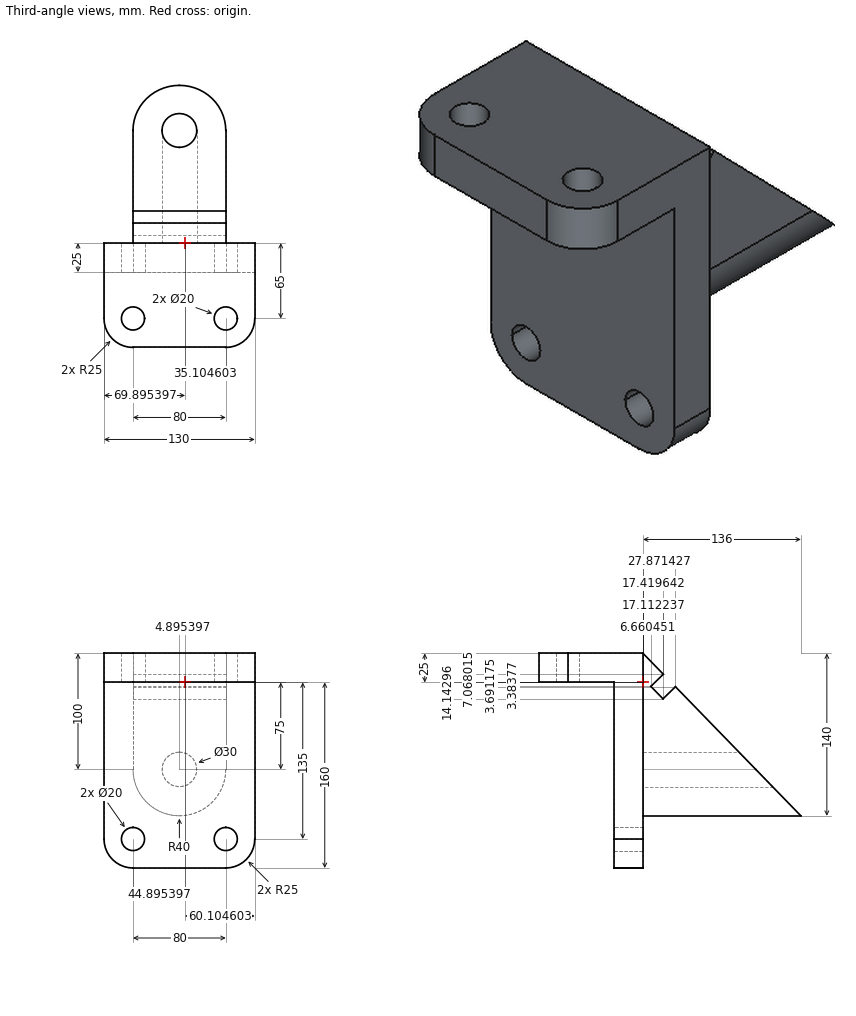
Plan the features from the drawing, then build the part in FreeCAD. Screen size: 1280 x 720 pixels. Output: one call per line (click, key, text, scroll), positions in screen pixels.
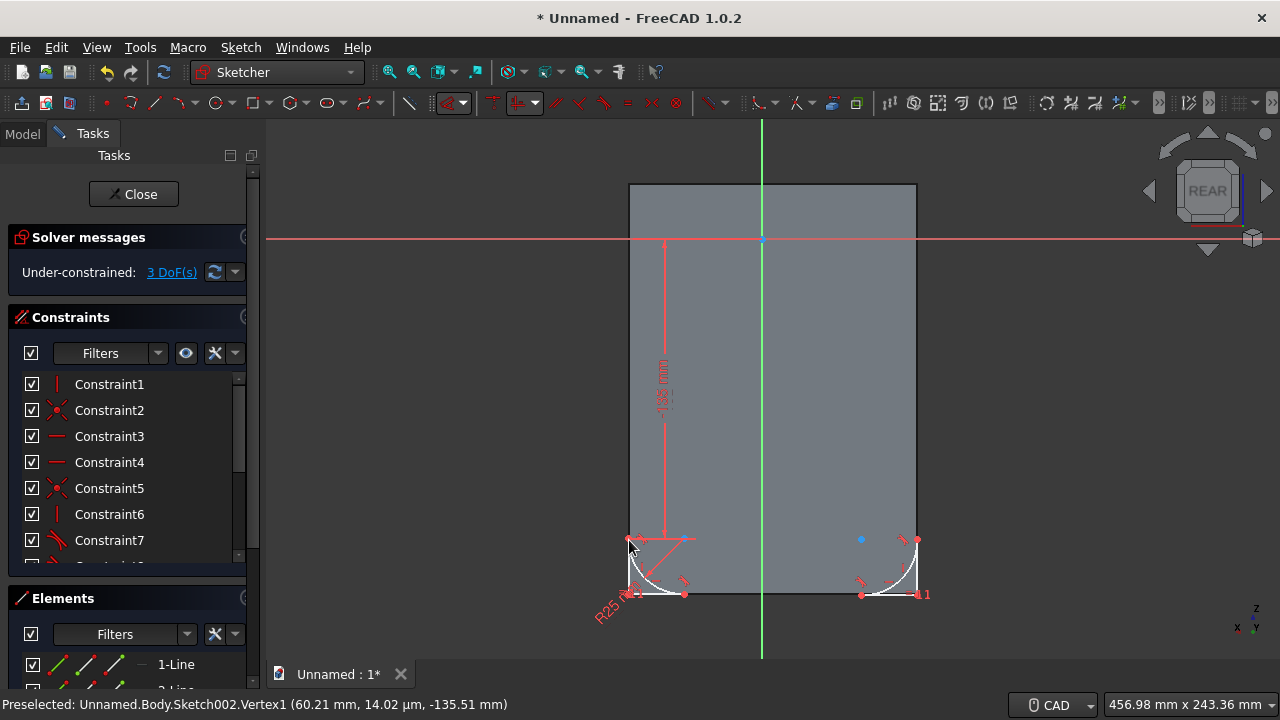
click(862, 595)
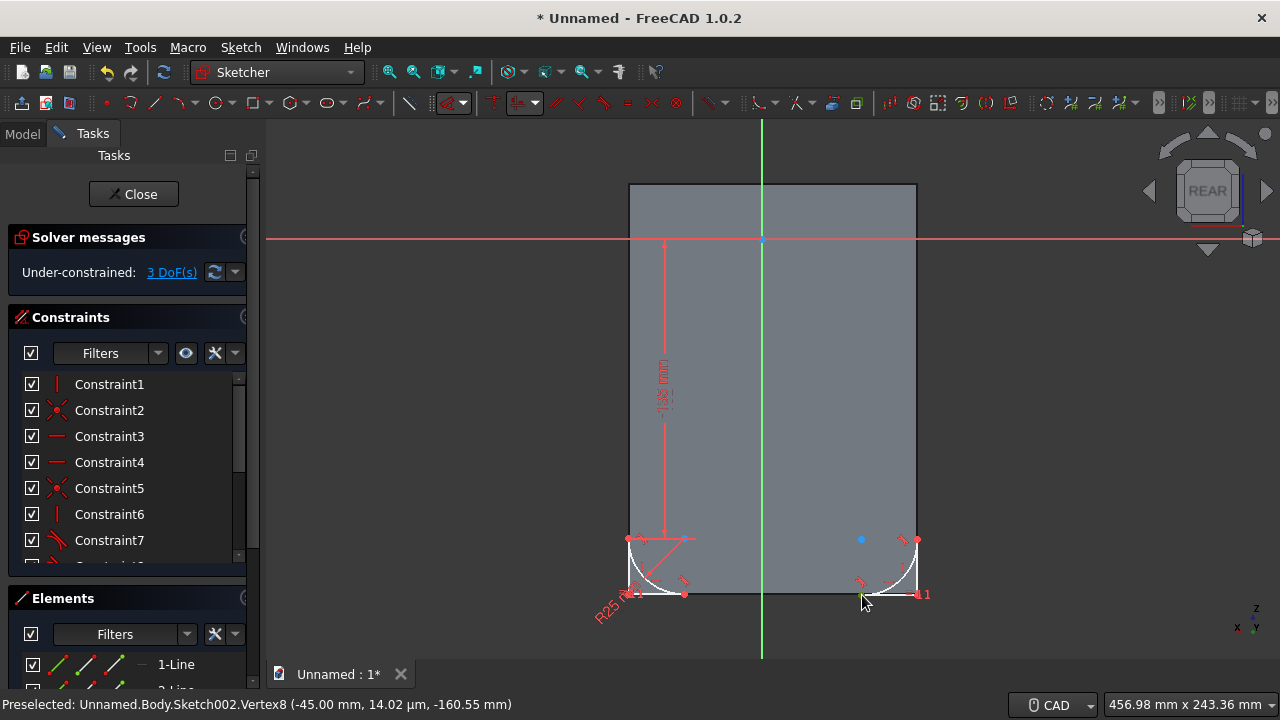
key(i)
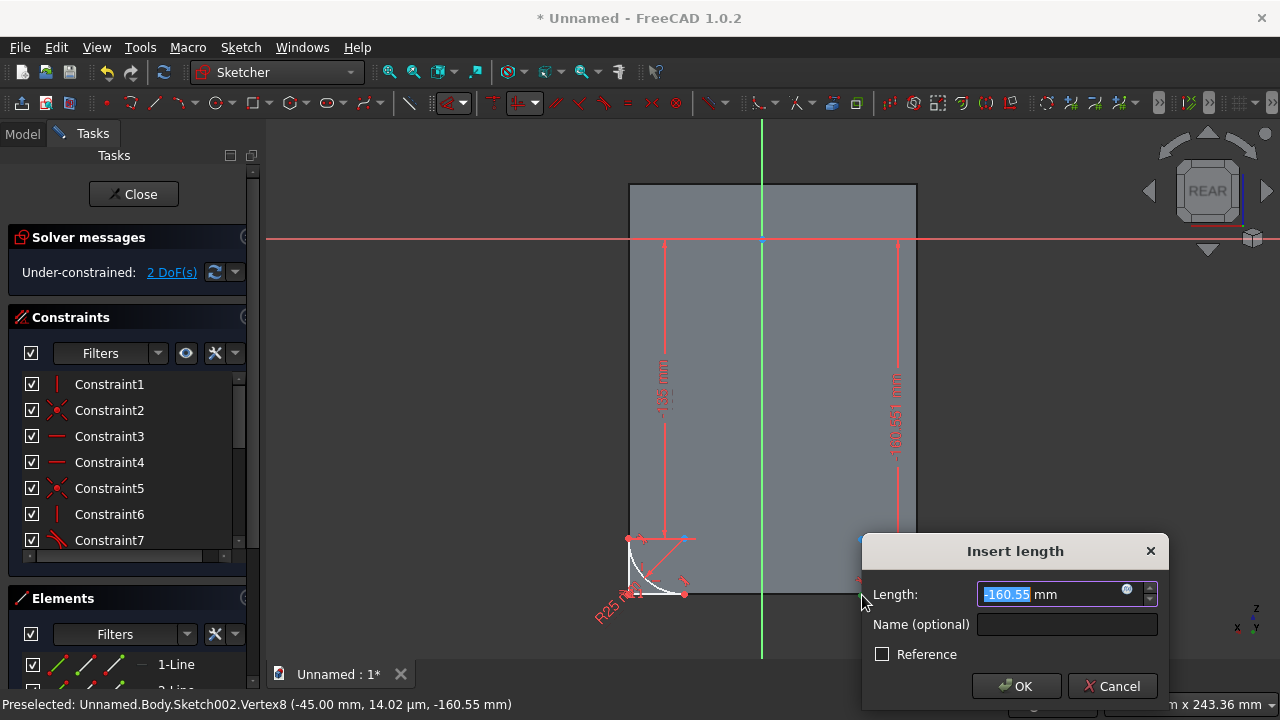
text(-160)
key(Return)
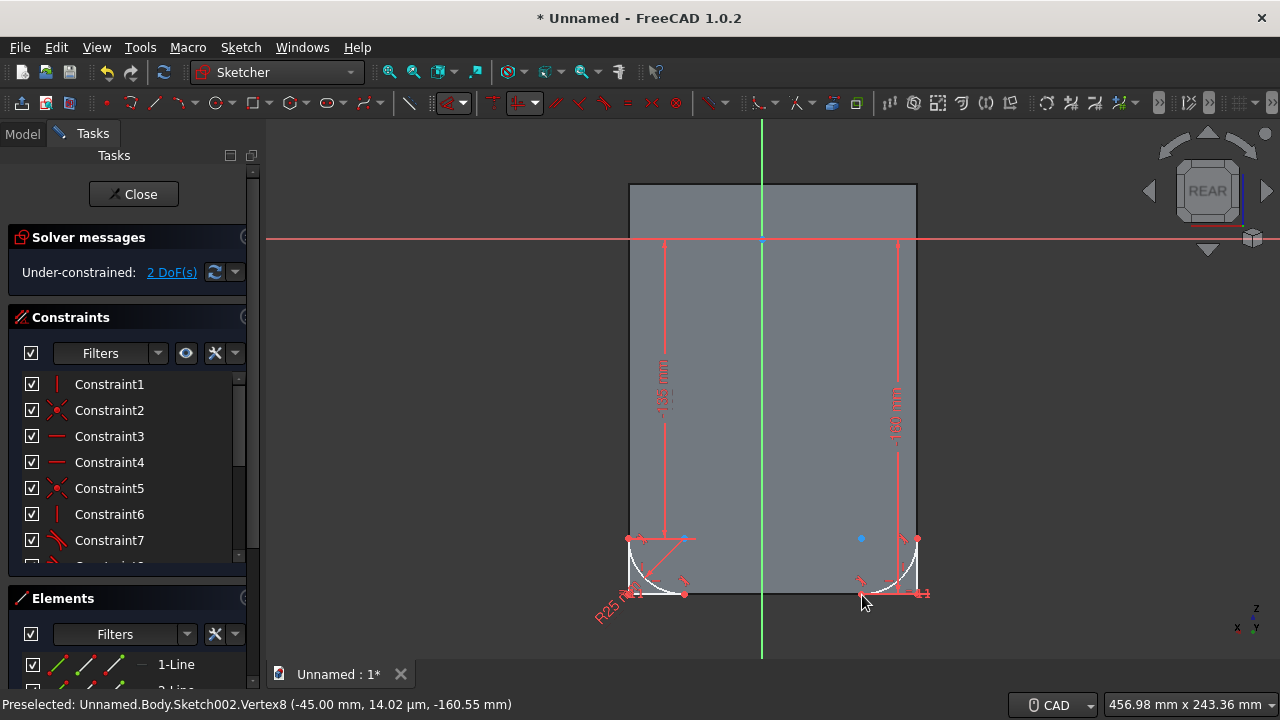
click(629, 539)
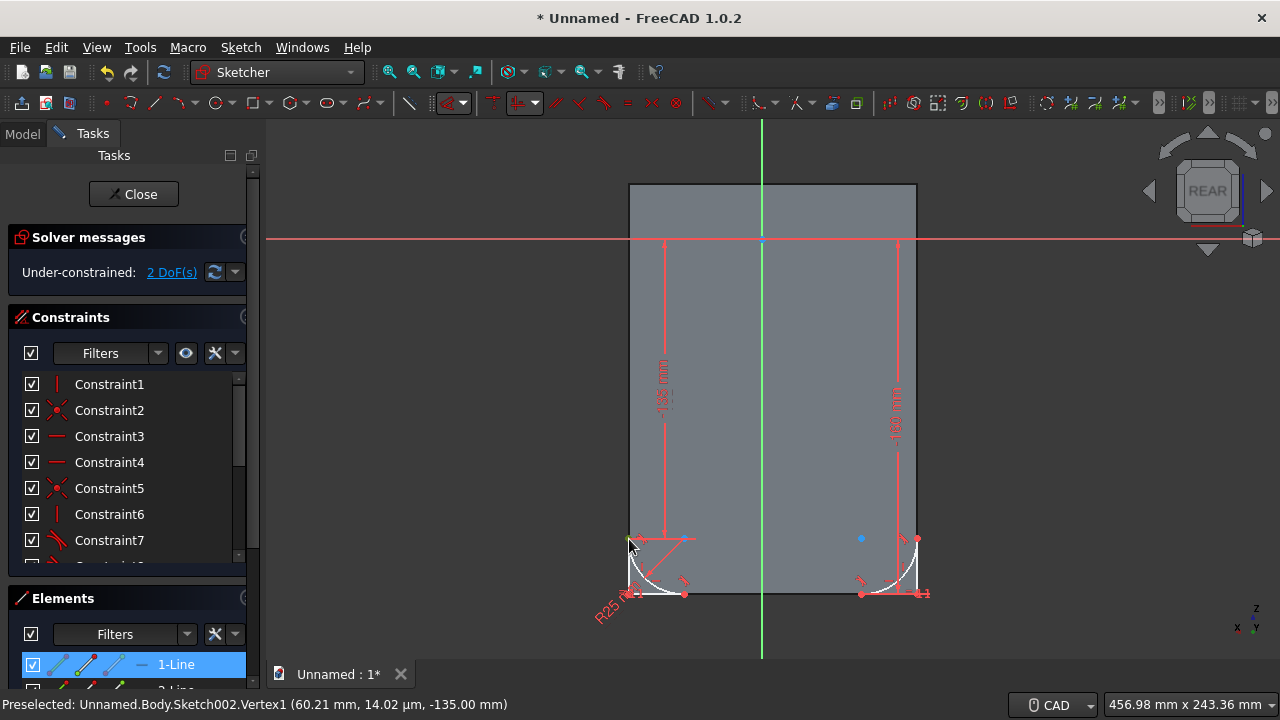
click(466, 104)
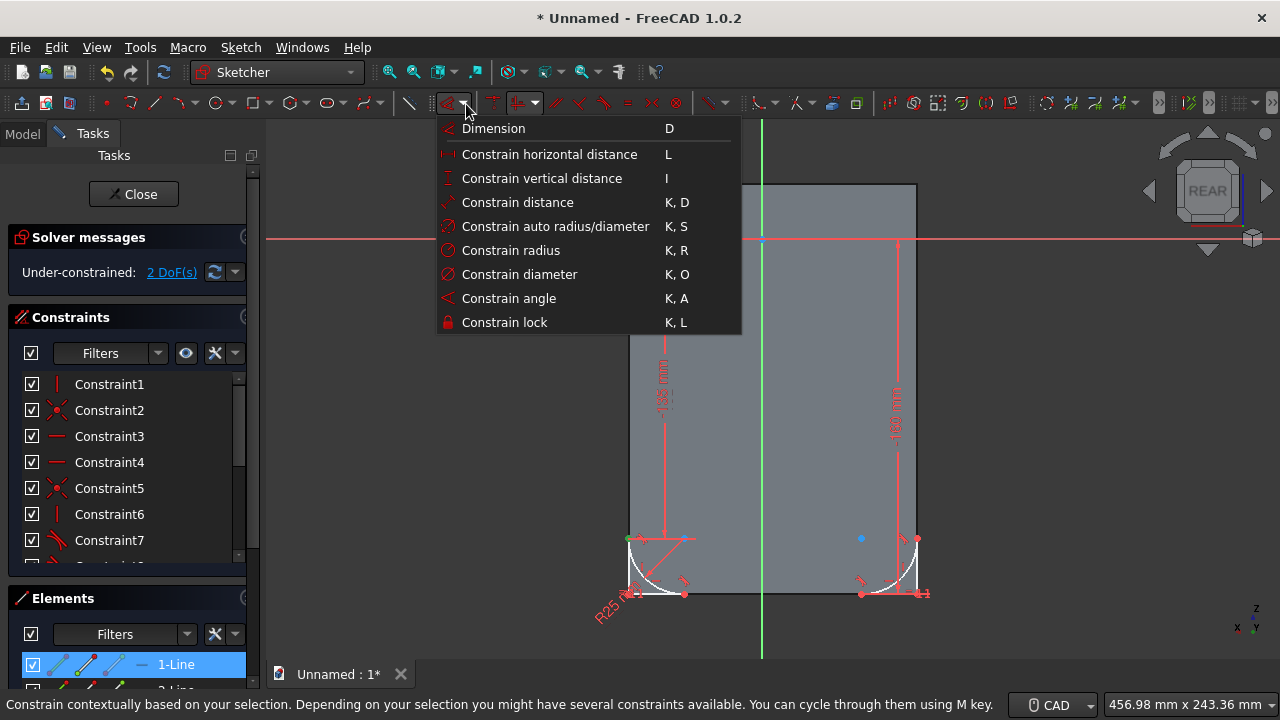
click(589, 154)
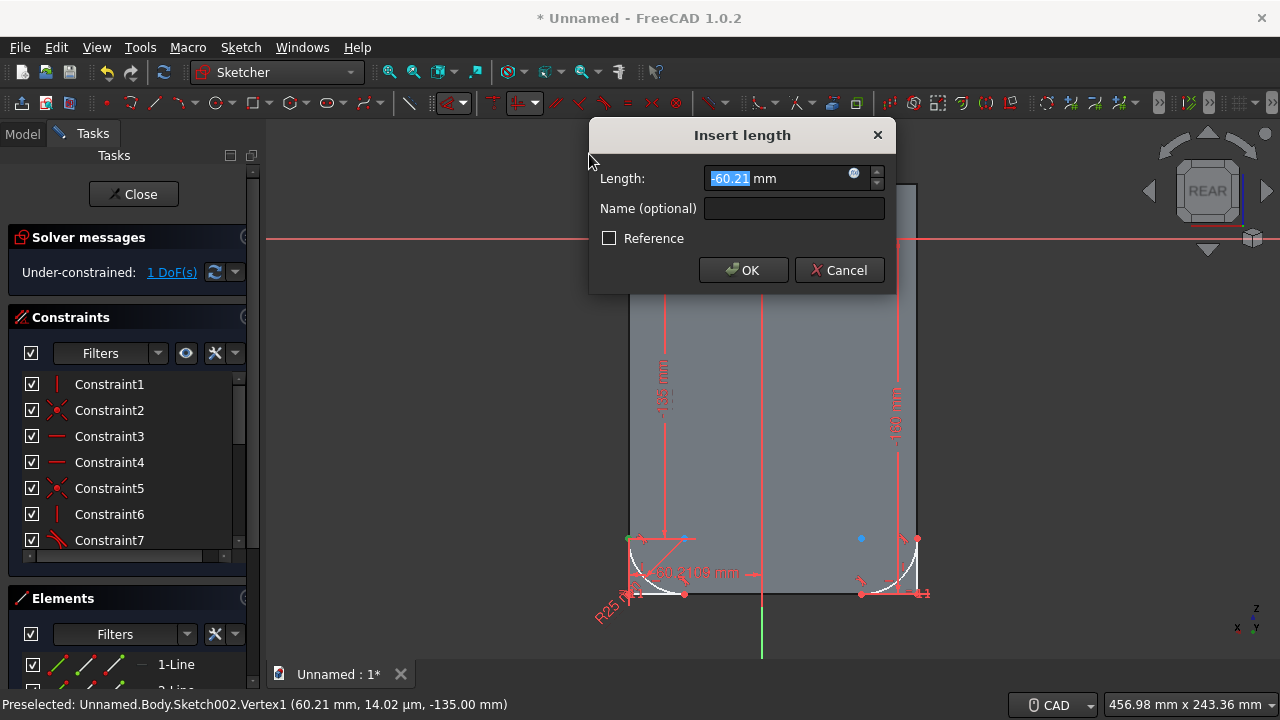
text(-60.104603)
key(Return)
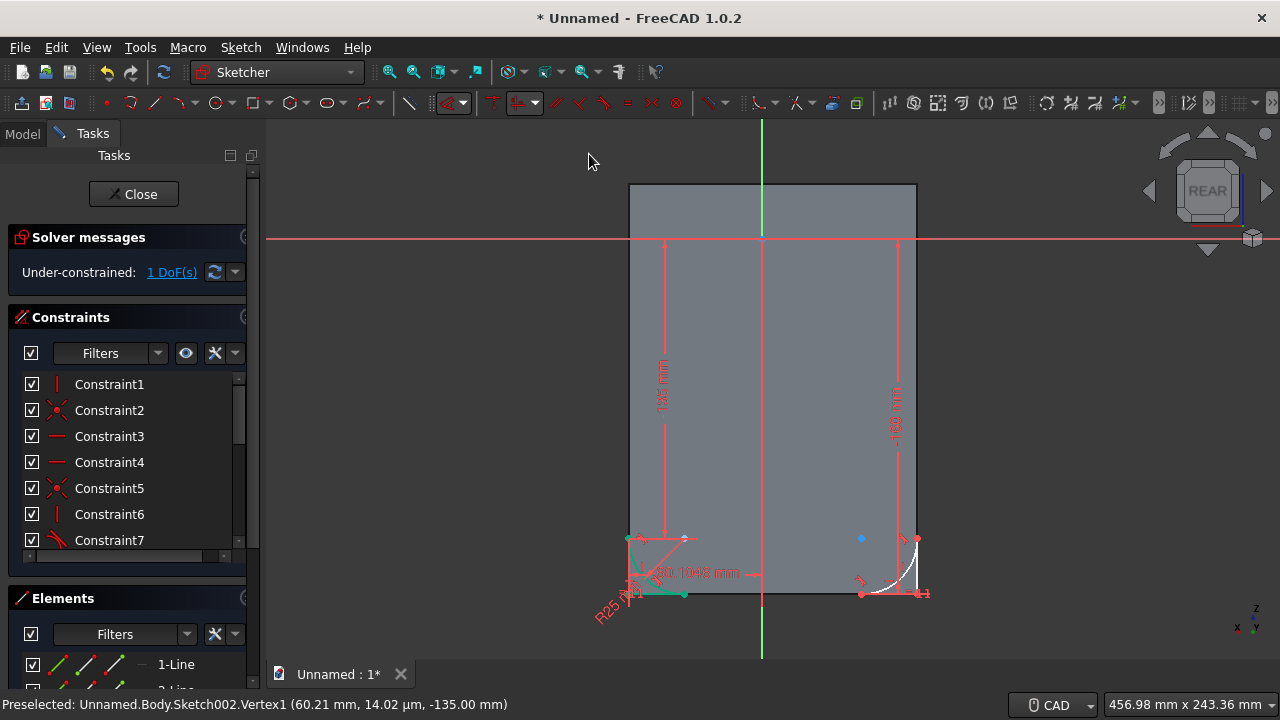
click(862, 594)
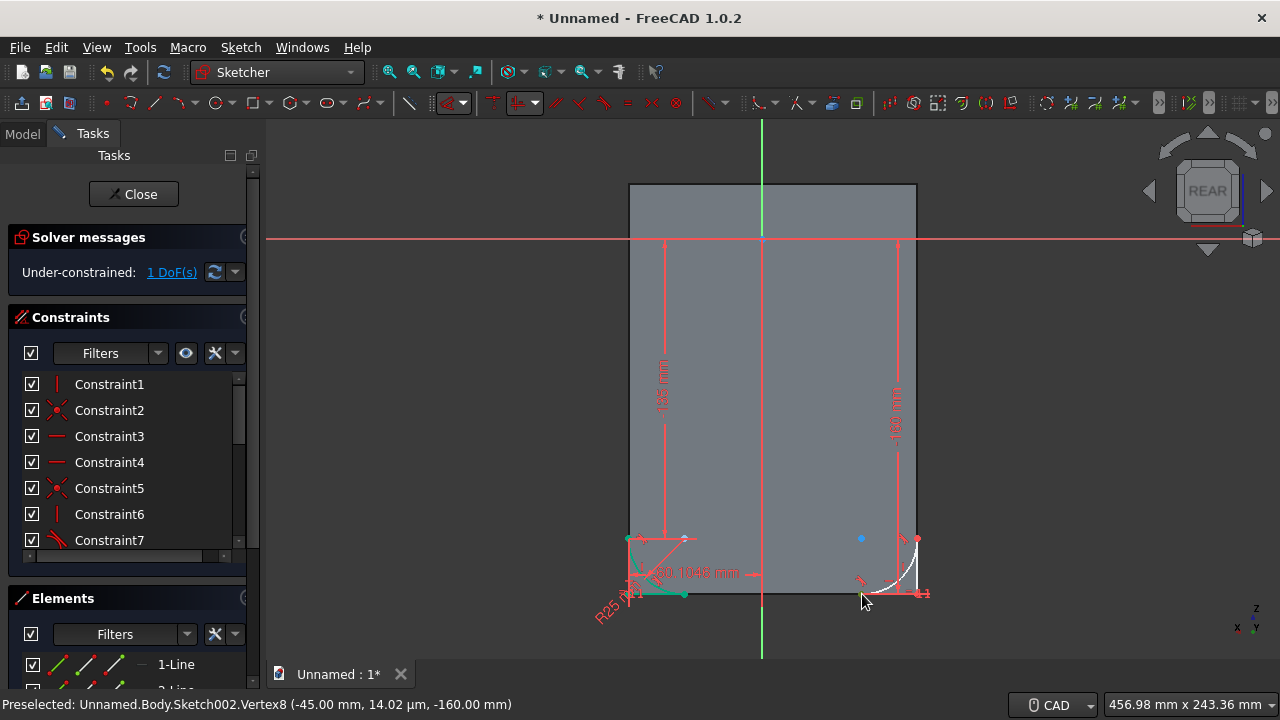
key(l)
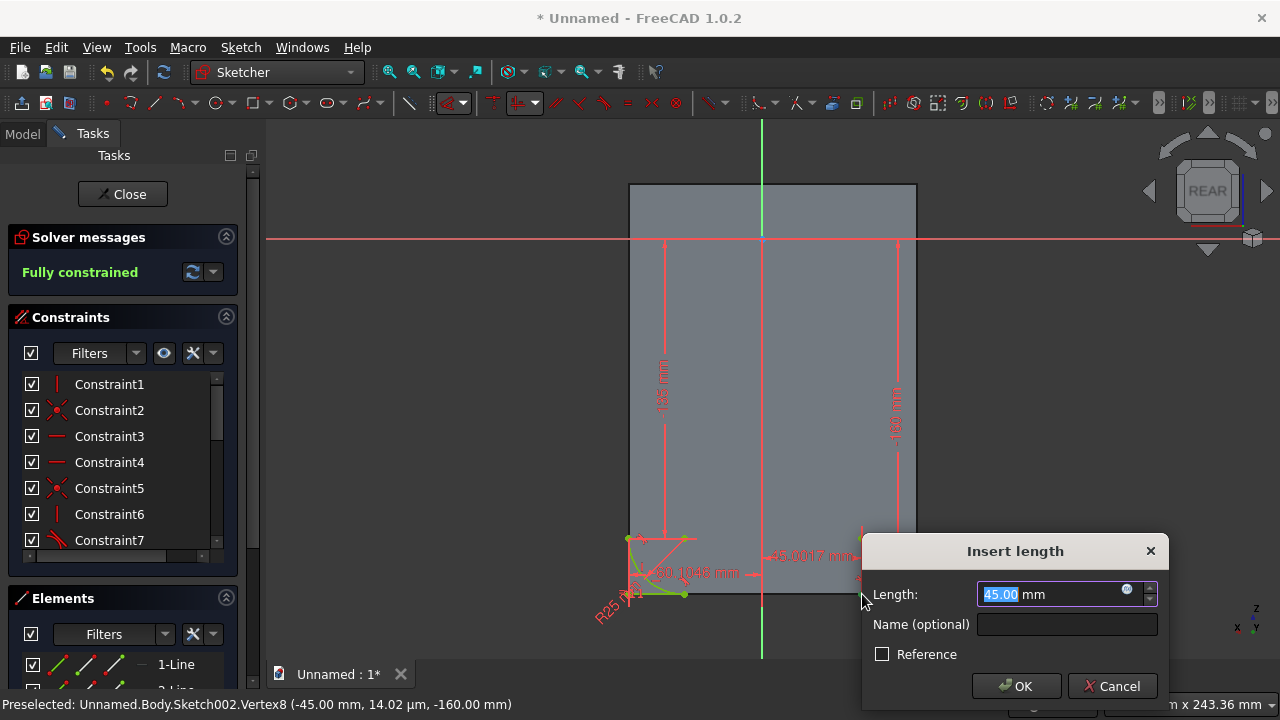
text(44.895397)
key(Return)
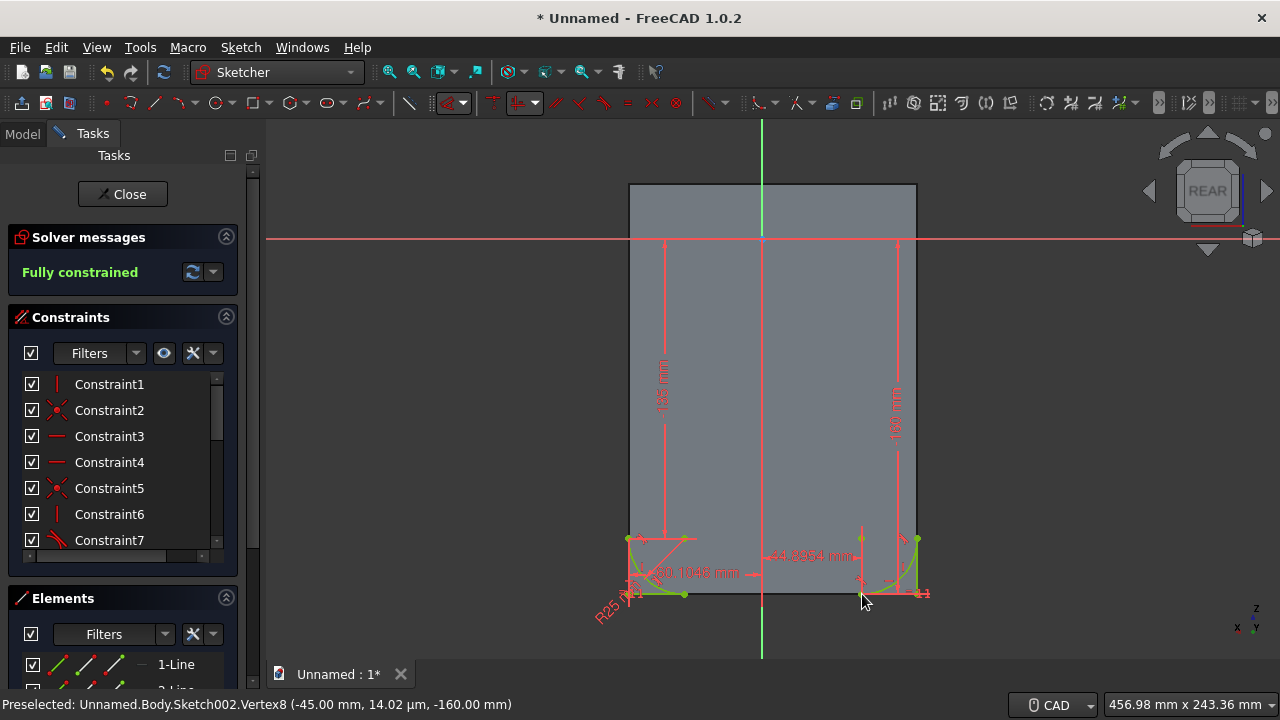
click(123, 194)